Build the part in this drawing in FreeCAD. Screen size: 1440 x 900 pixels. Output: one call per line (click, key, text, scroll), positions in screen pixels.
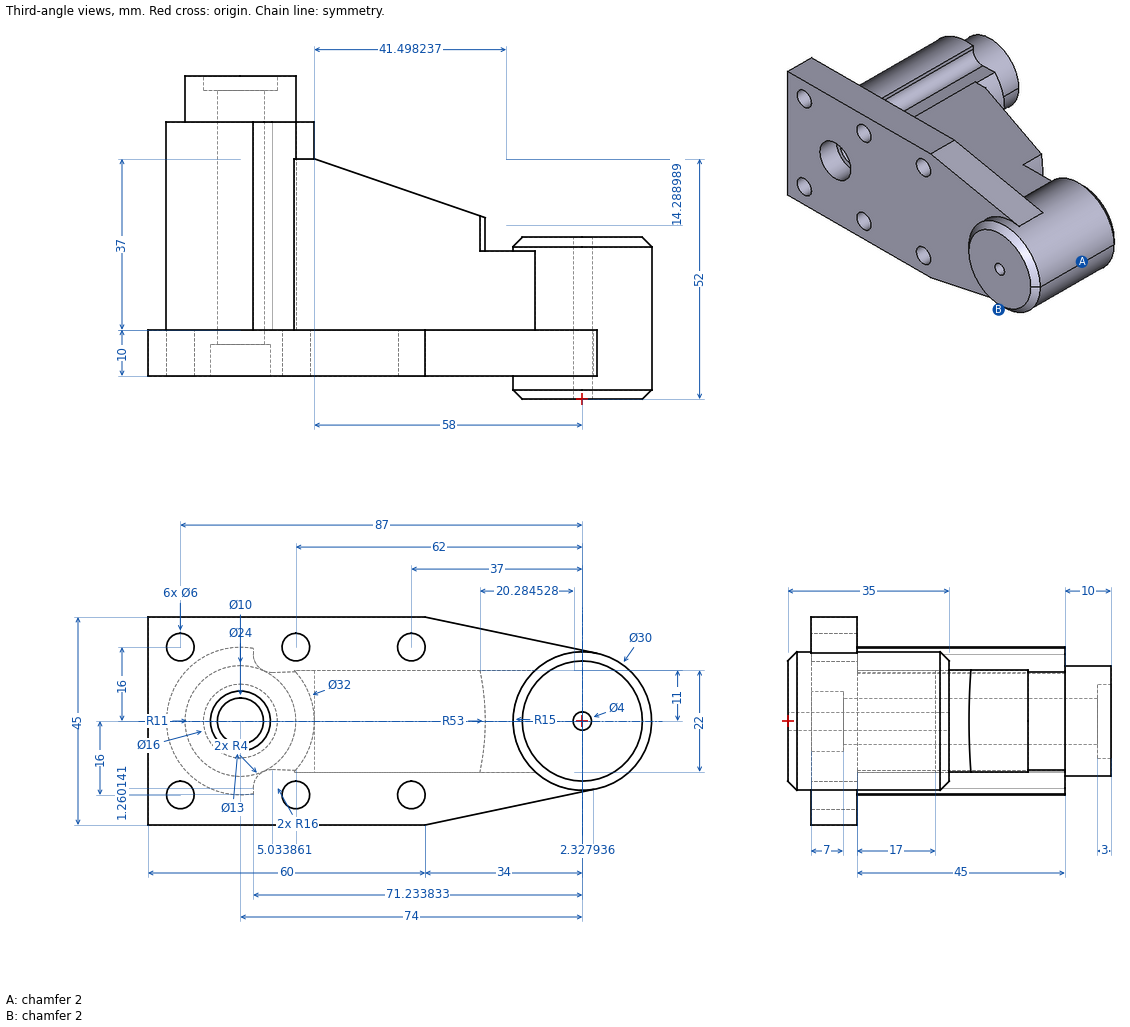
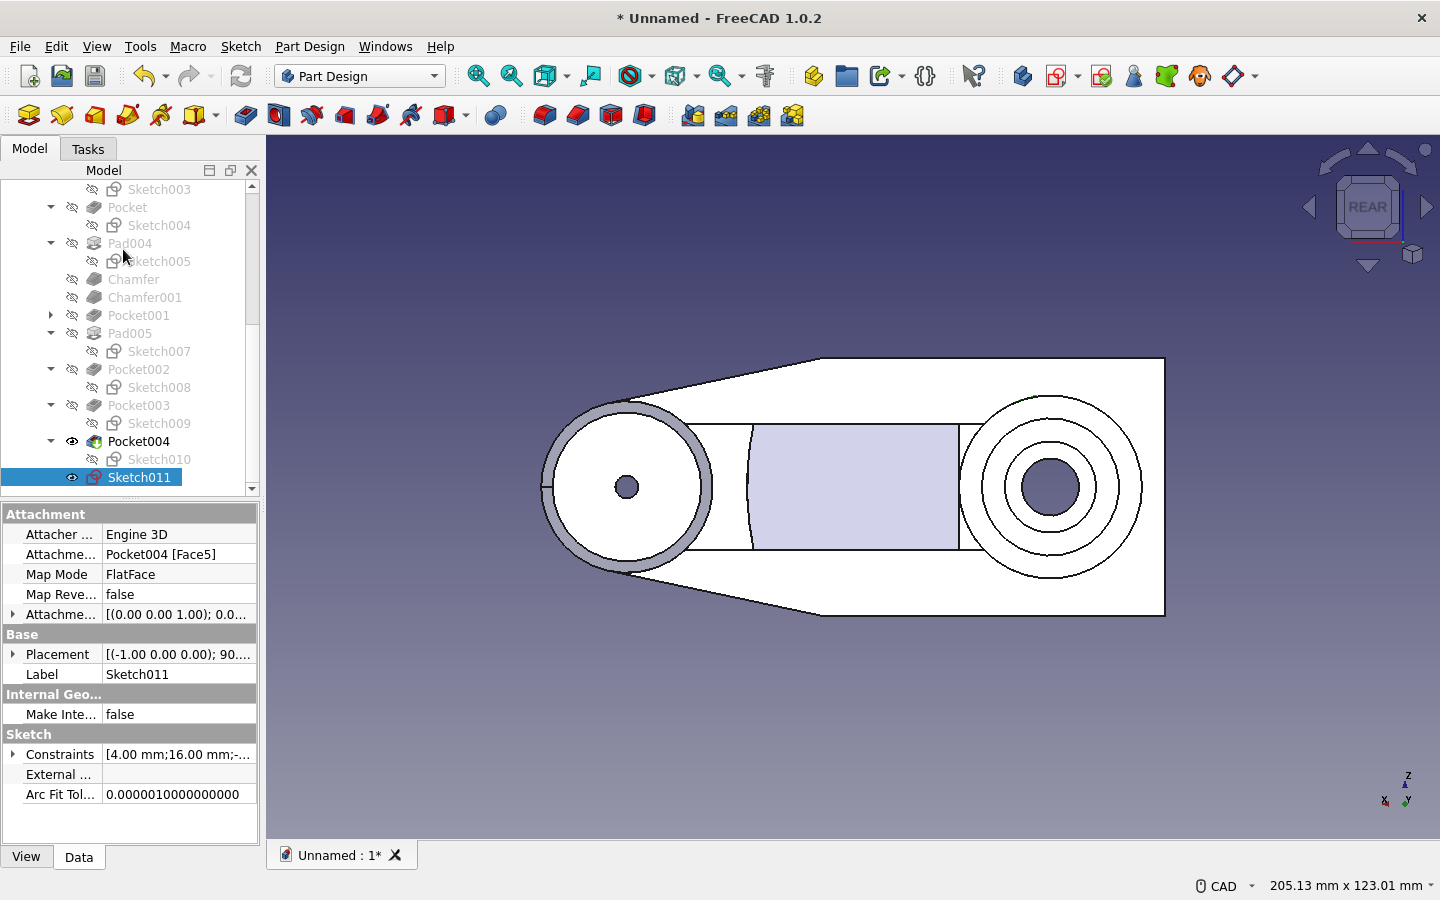
click(246, 116)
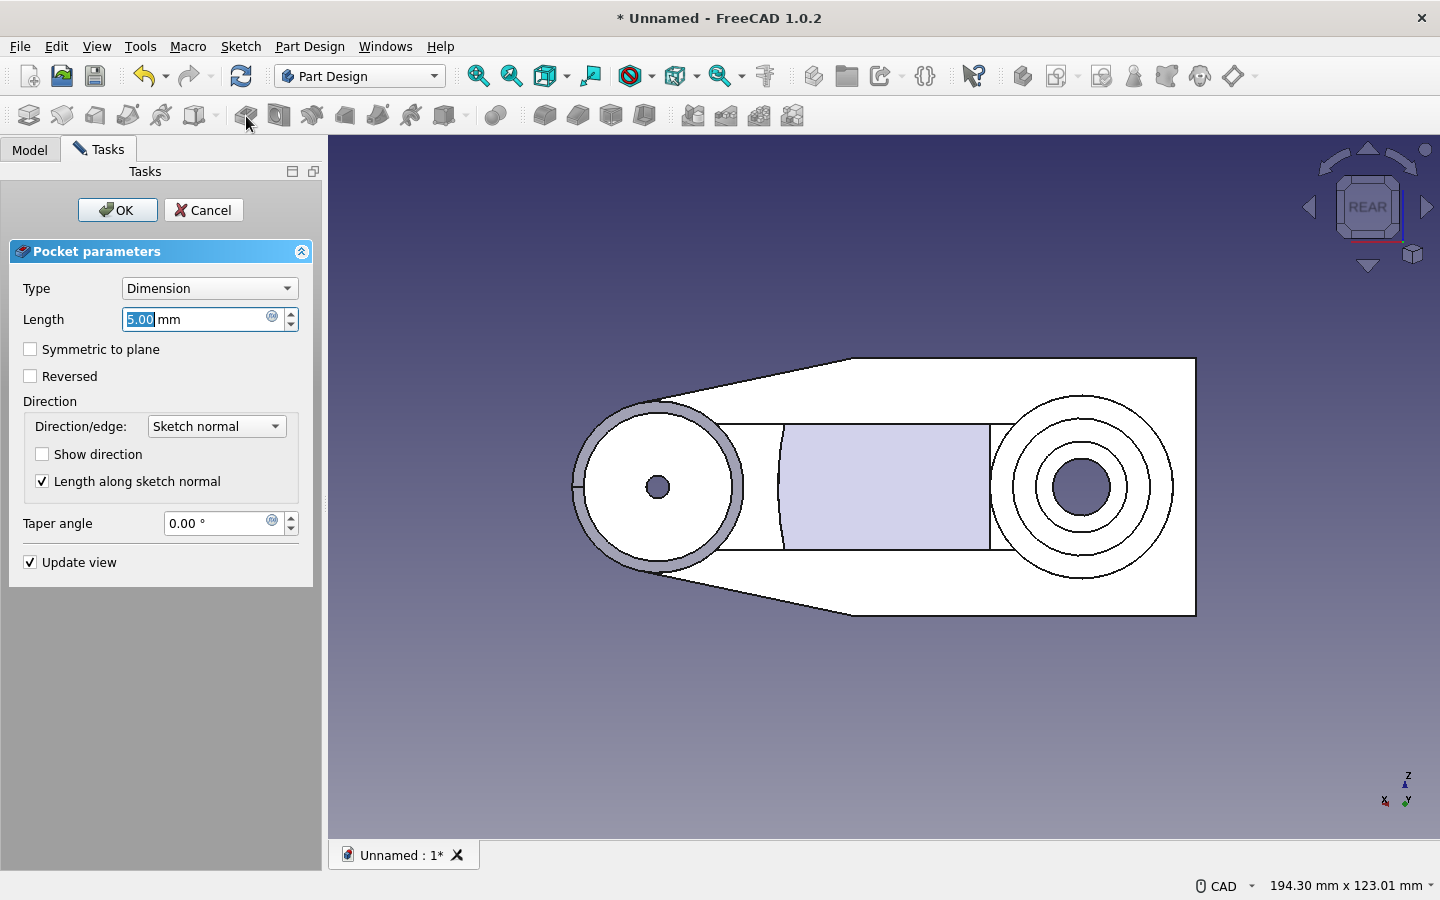
text(45)
key(Tab)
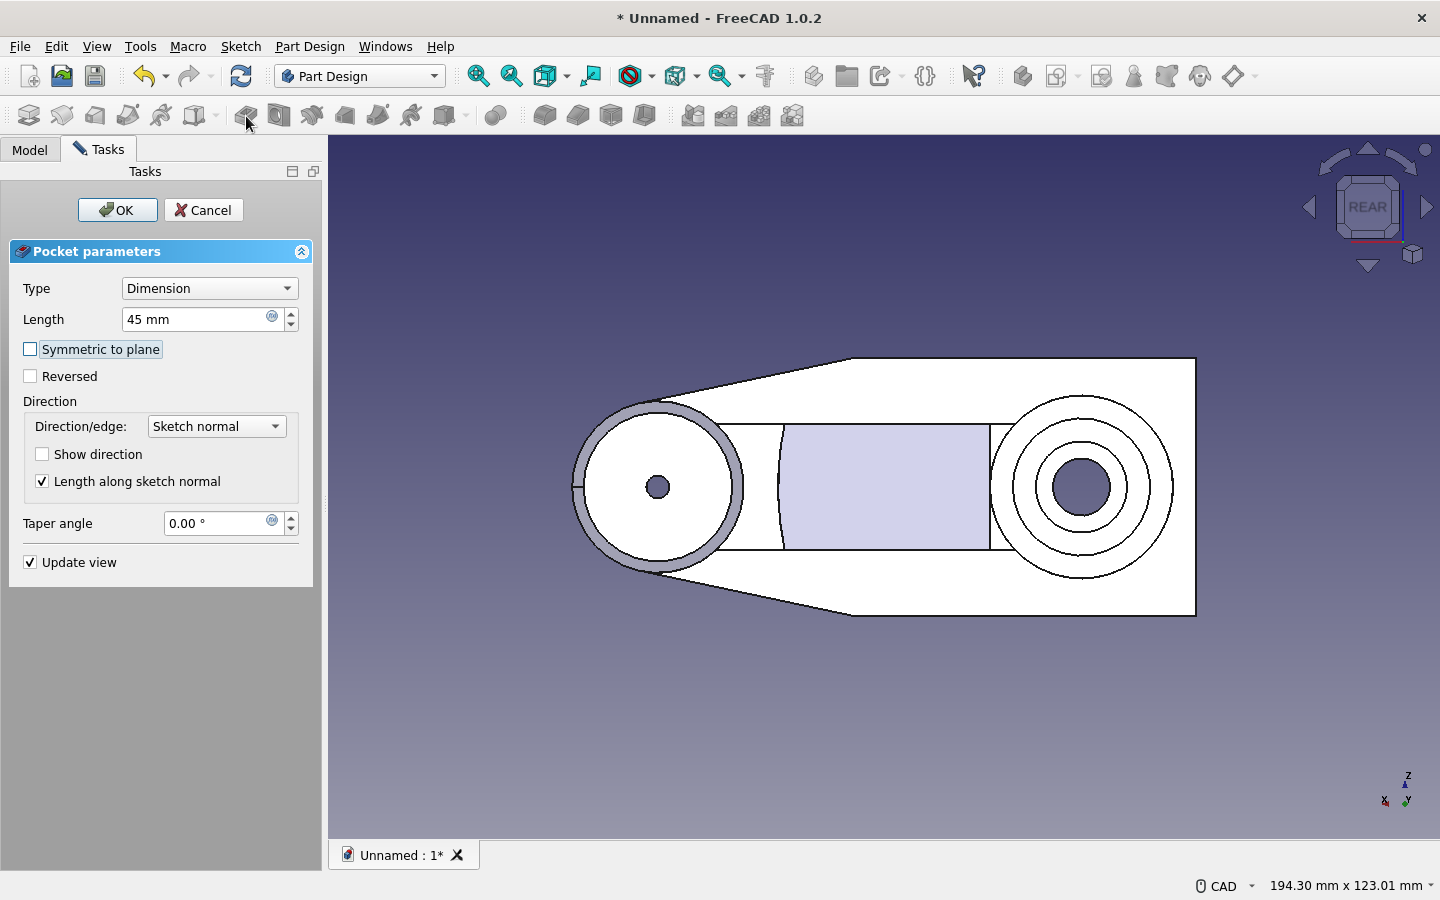
click(31, 376)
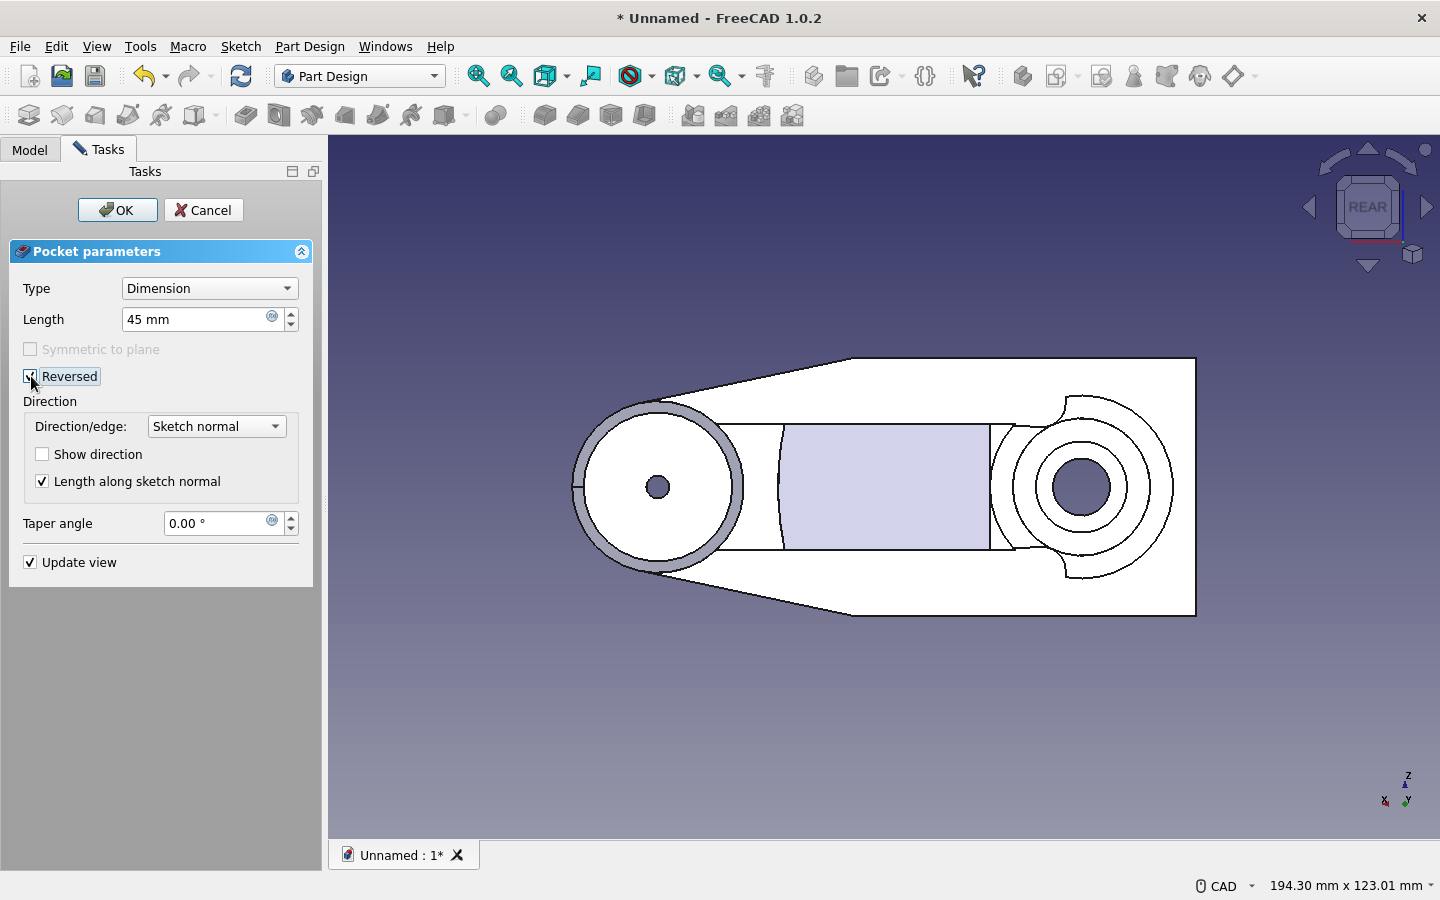
click(118, 210)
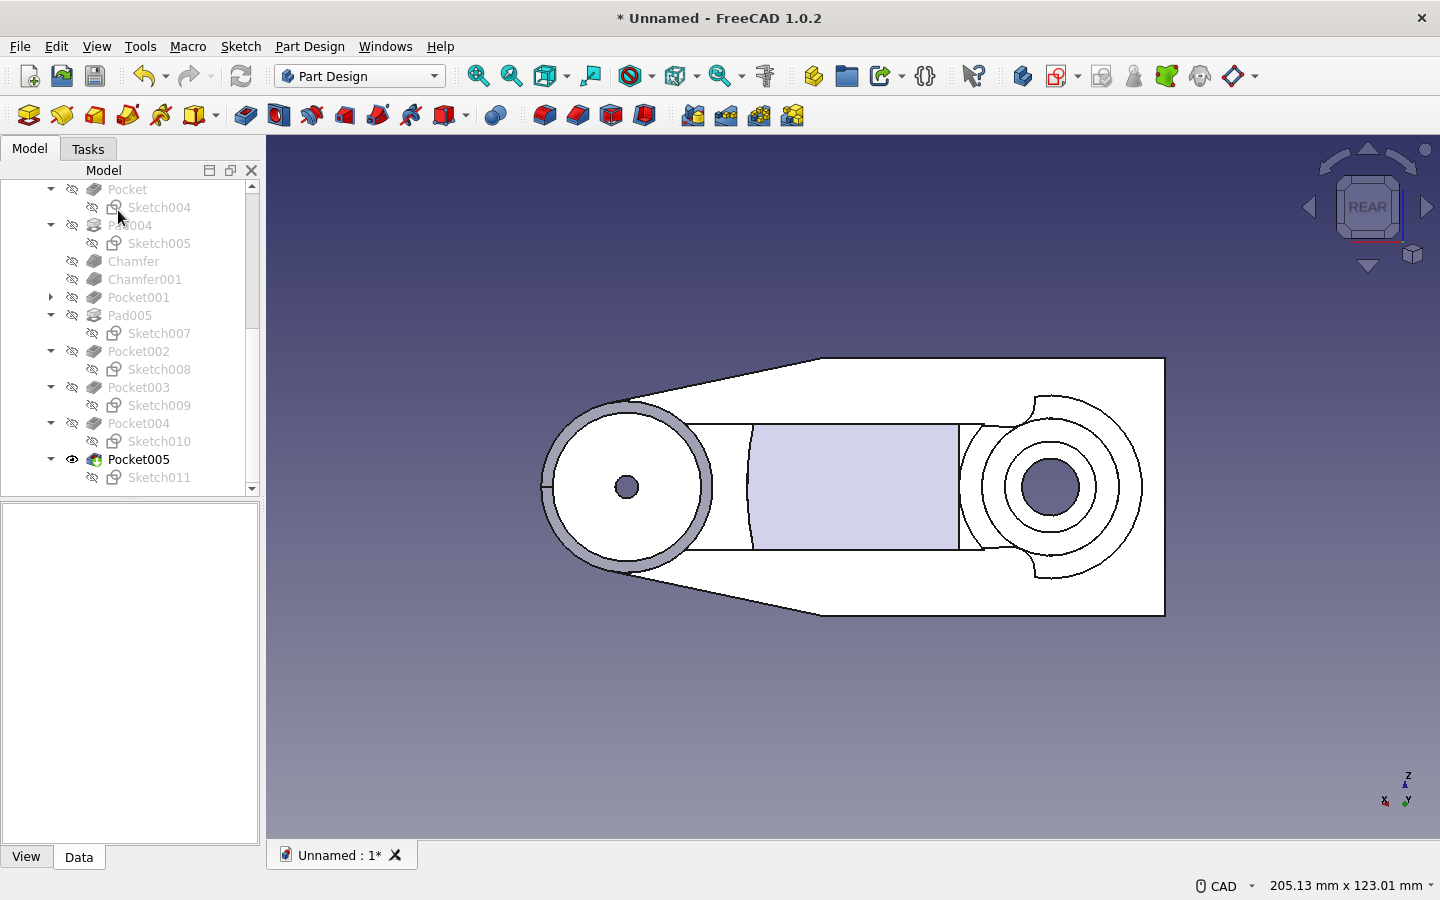
click(887, 376)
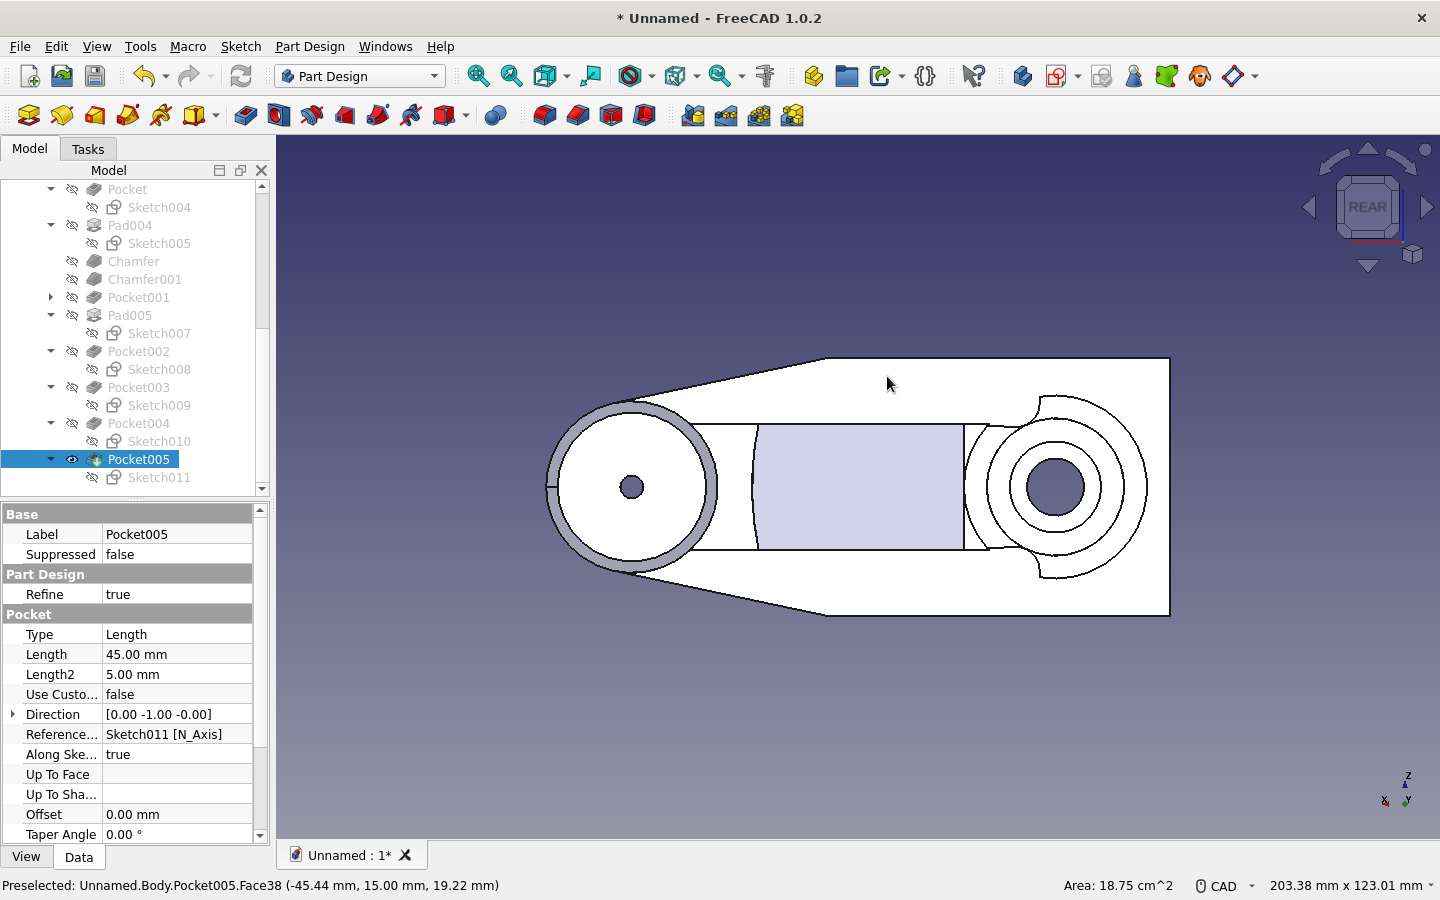
click(1056, 76)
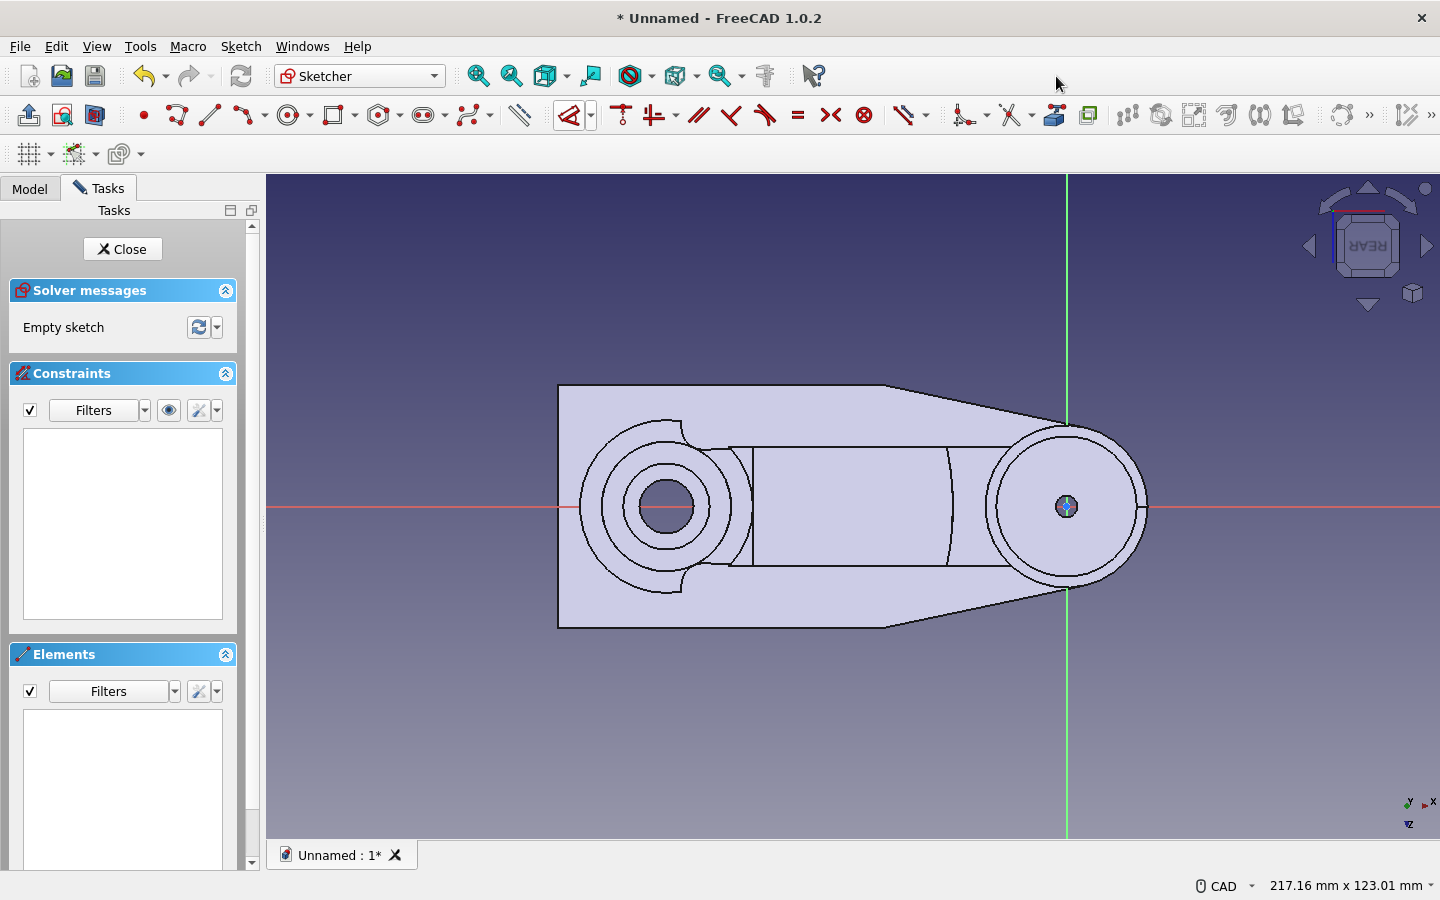
scroll(902, 506, up, 2)